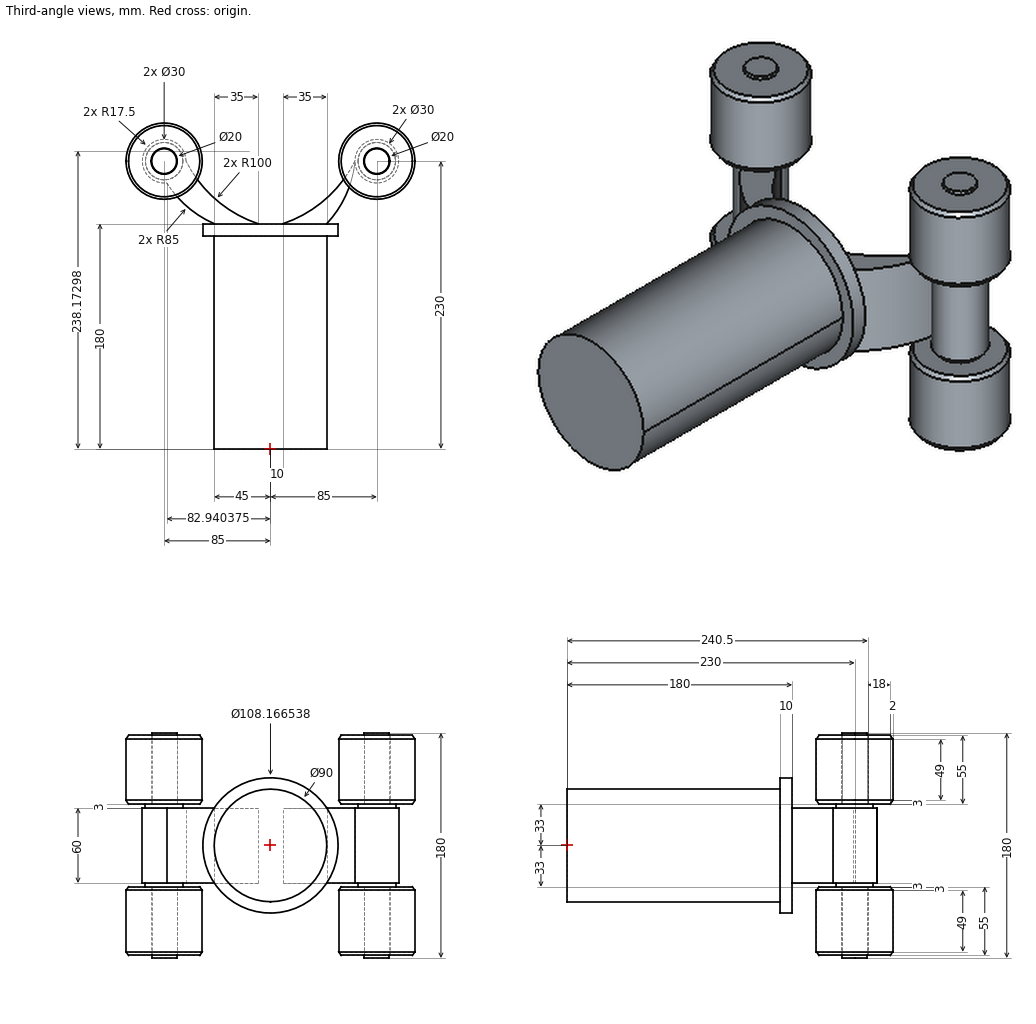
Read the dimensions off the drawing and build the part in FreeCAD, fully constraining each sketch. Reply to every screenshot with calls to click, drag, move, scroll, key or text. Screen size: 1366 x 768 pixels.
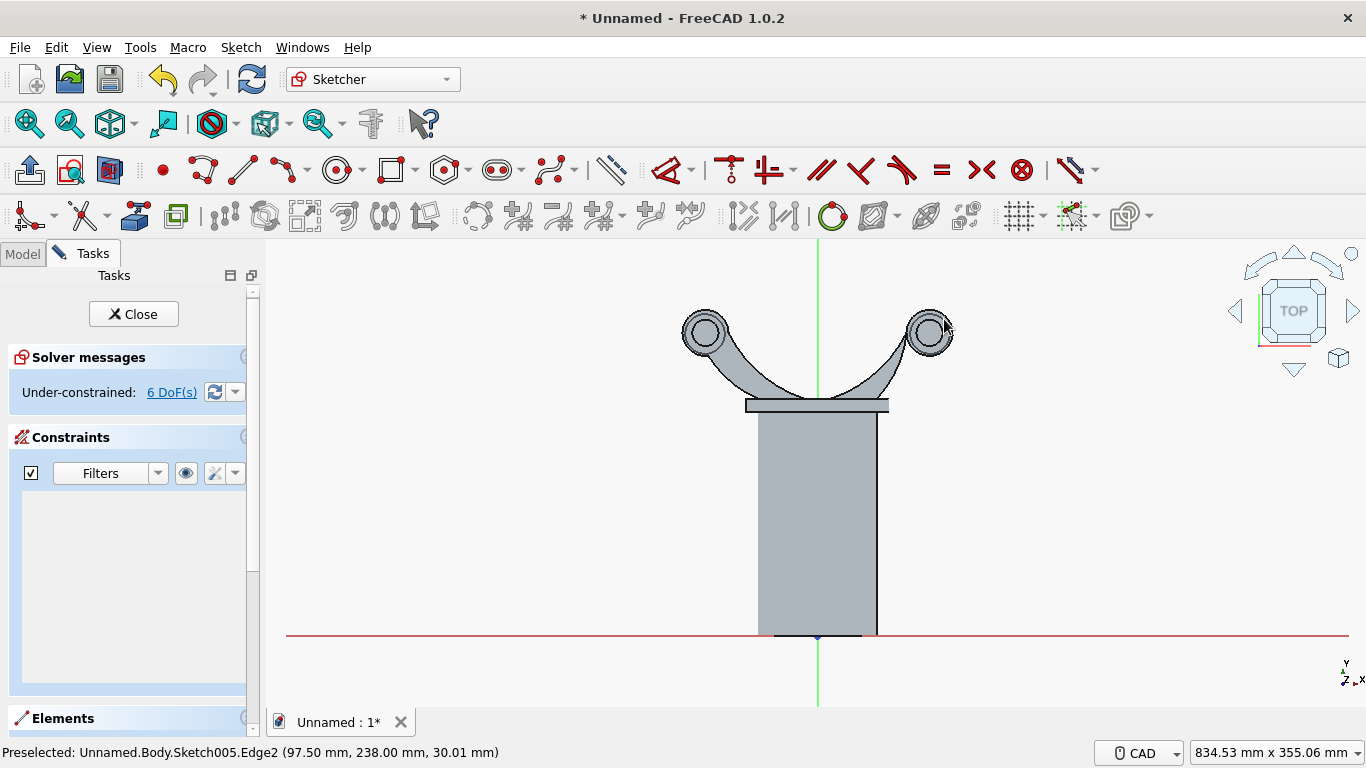
click(719, 320)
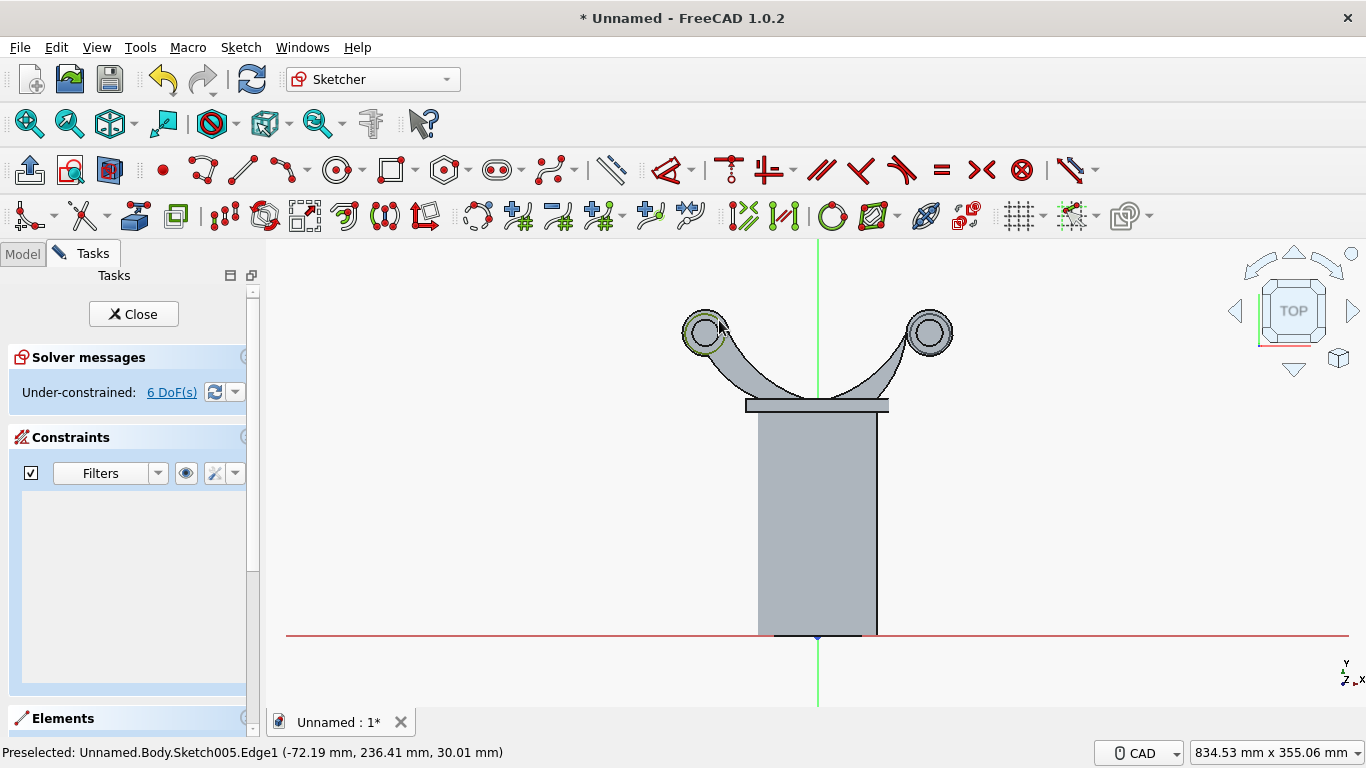
click(944, 320)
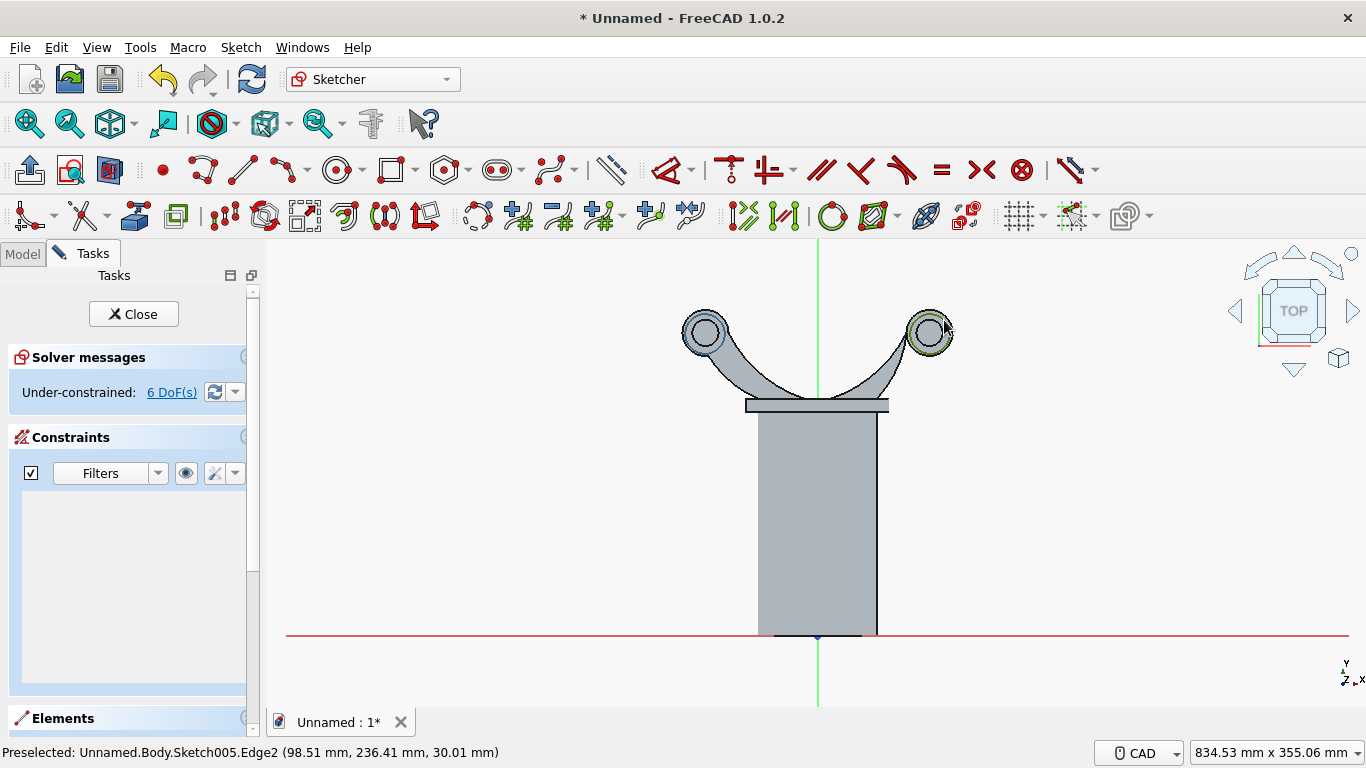
click(942, 170)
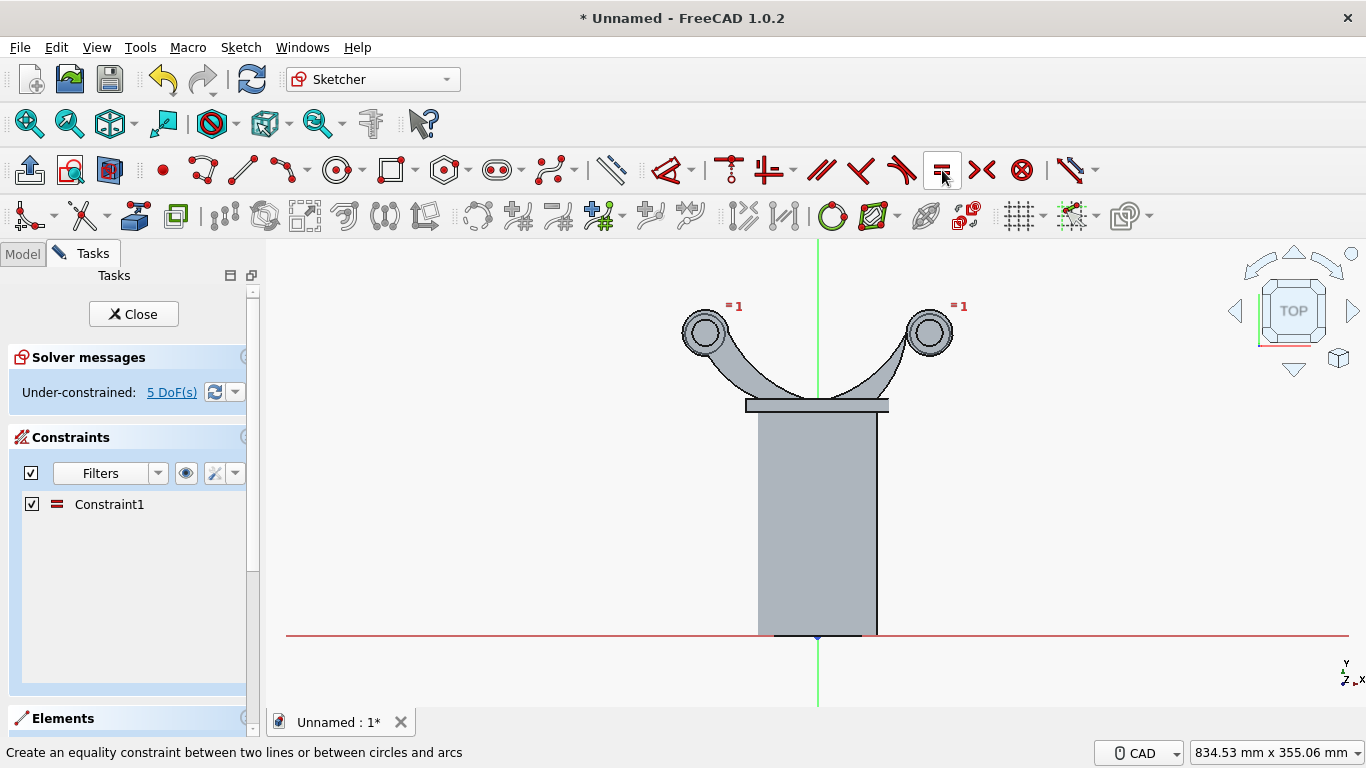
click(666, 170)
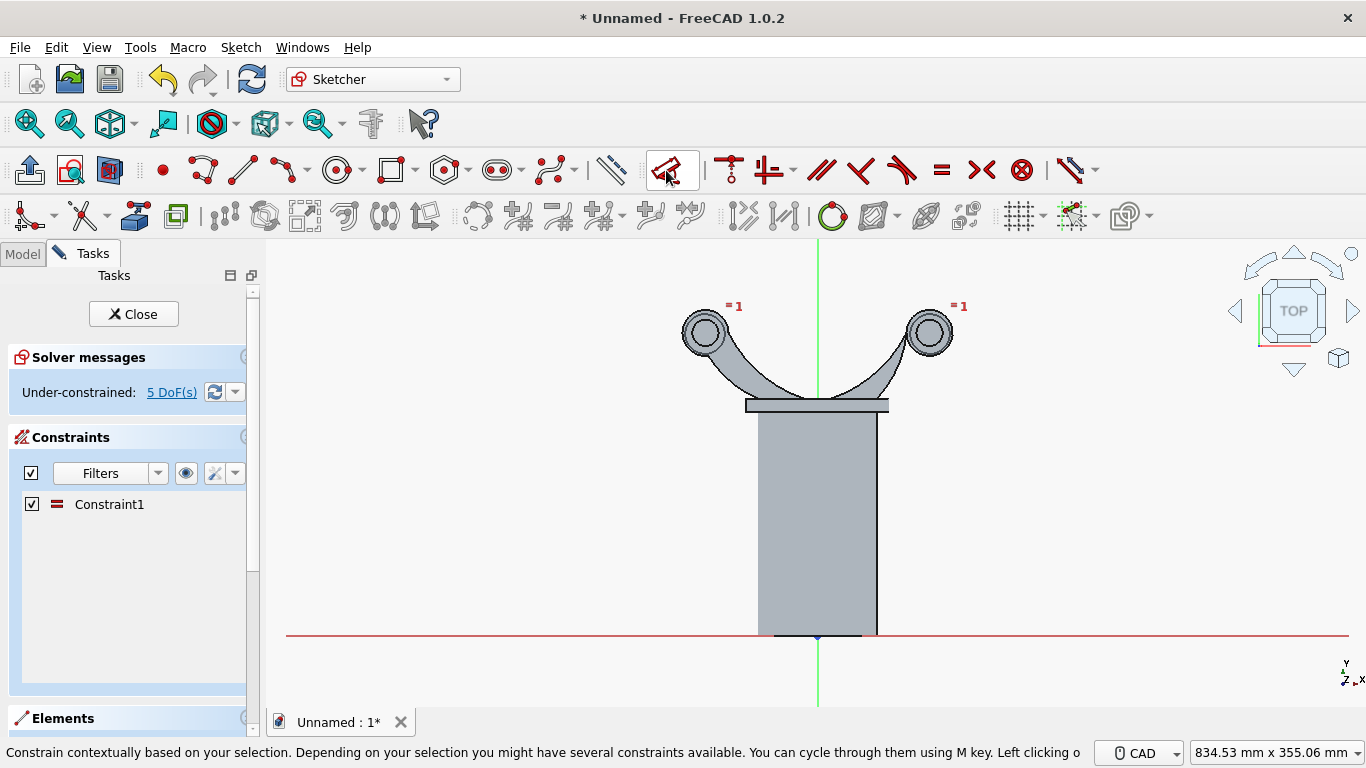
click(719, 320)
click(742, 297)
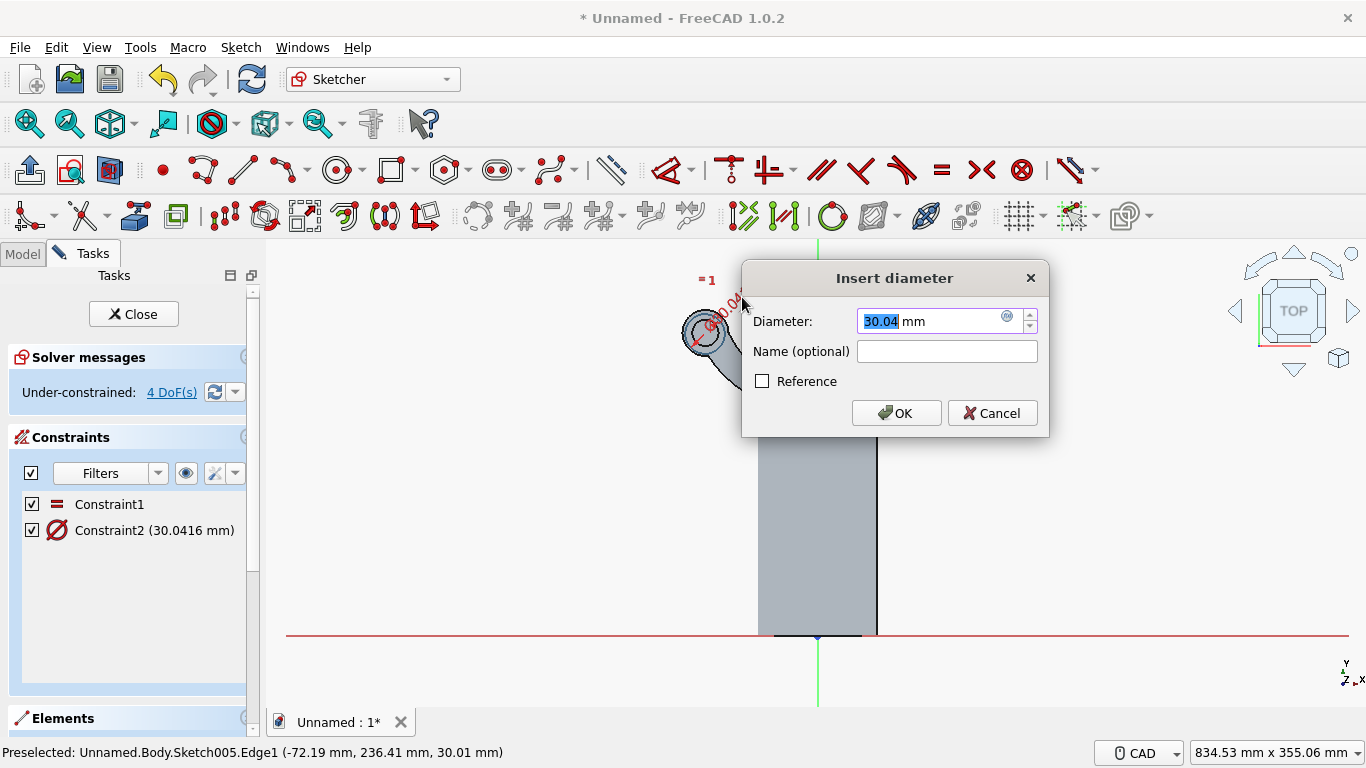
text(30)
key(Return)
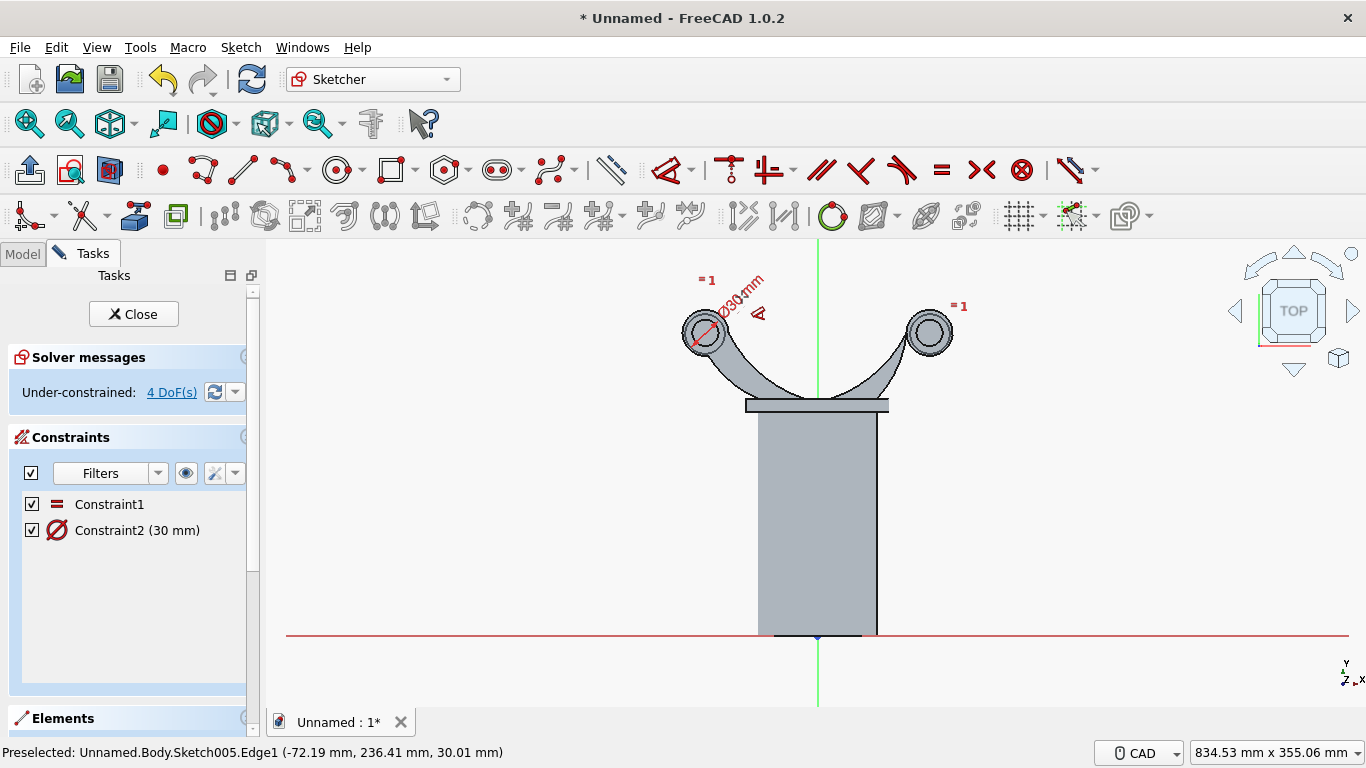
click(705, 334)
click(761, 670)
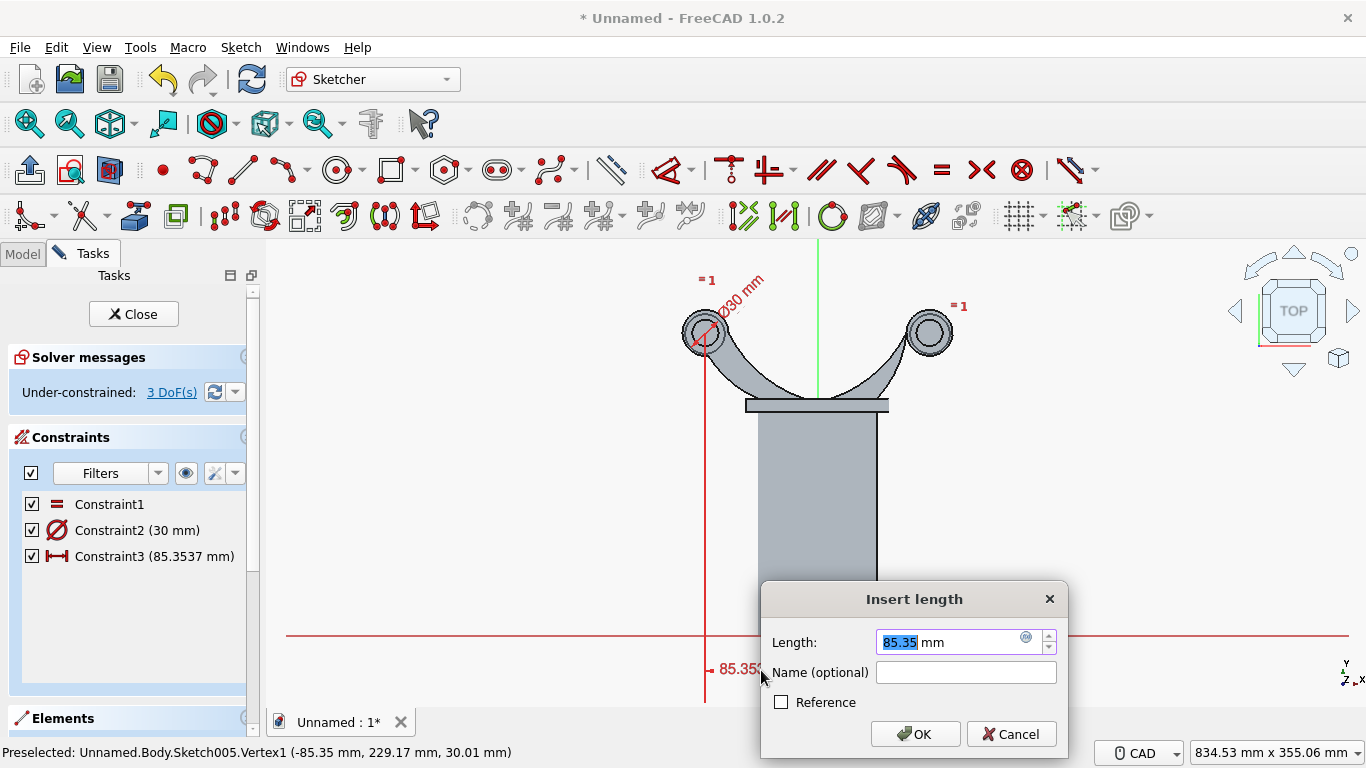
text(85)
key(Return)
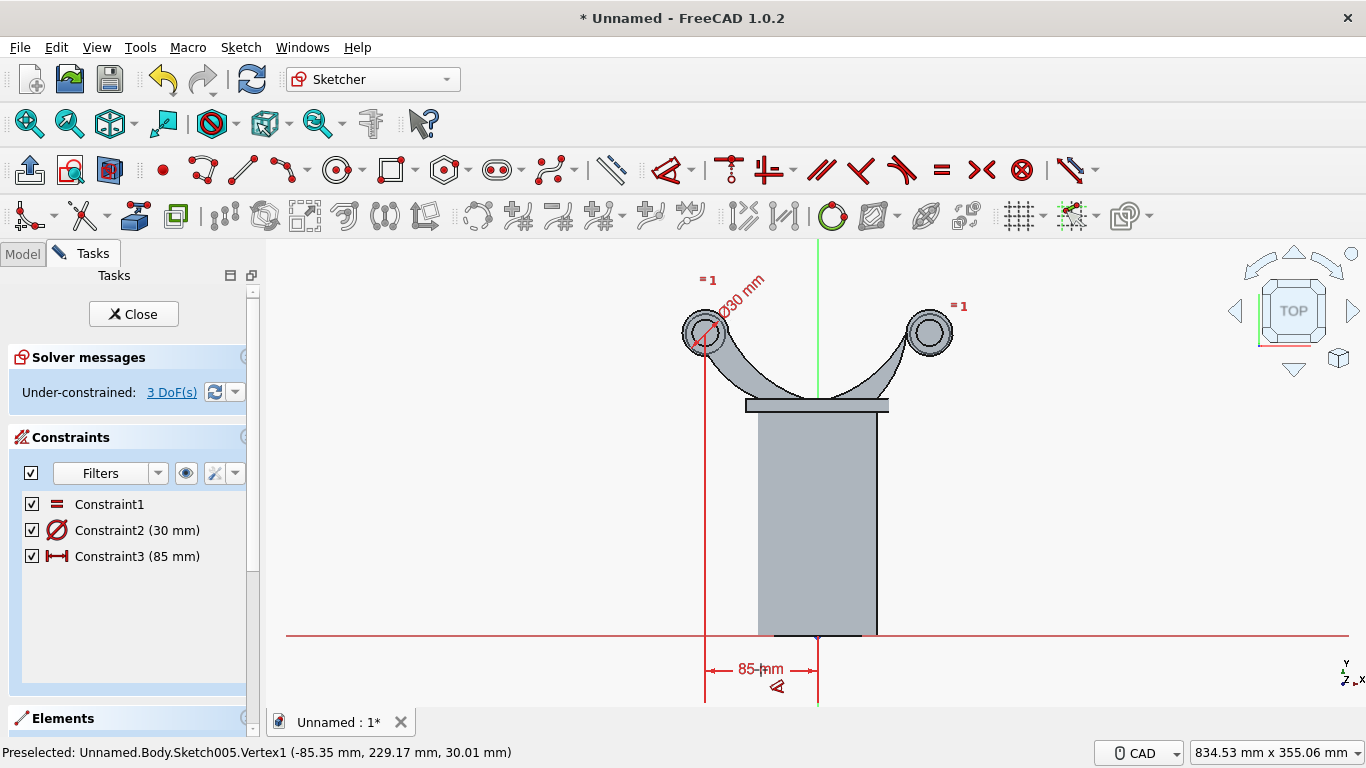
click(930, 334)
click(874, 670)